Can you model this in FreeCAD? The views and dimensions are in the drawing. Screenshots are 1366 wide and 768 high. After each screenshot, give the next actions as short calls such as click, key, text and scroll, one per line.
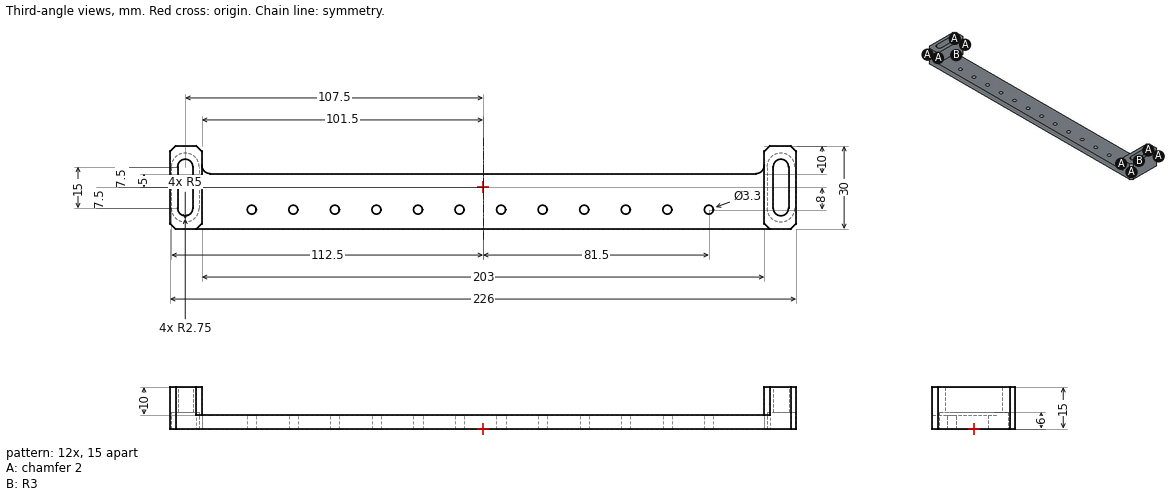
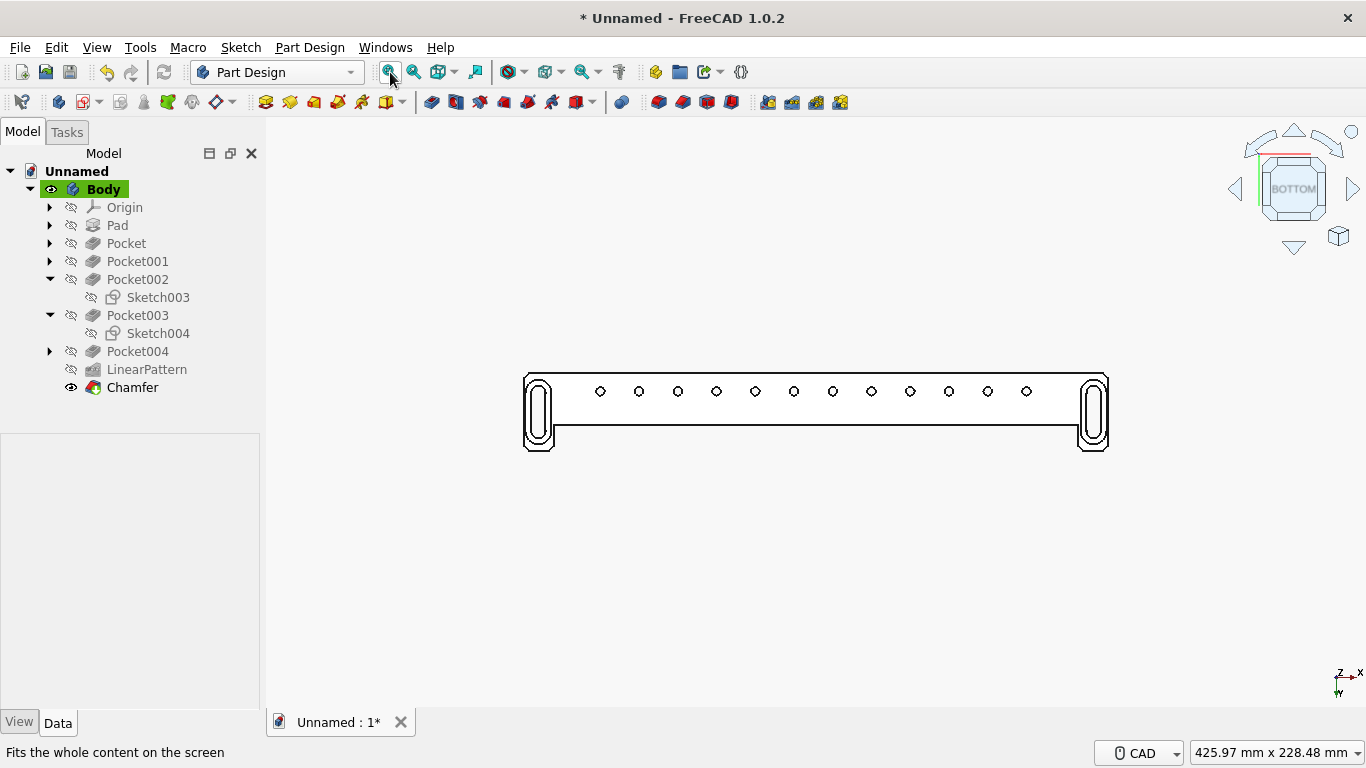
scroll(554, 424, up, 6)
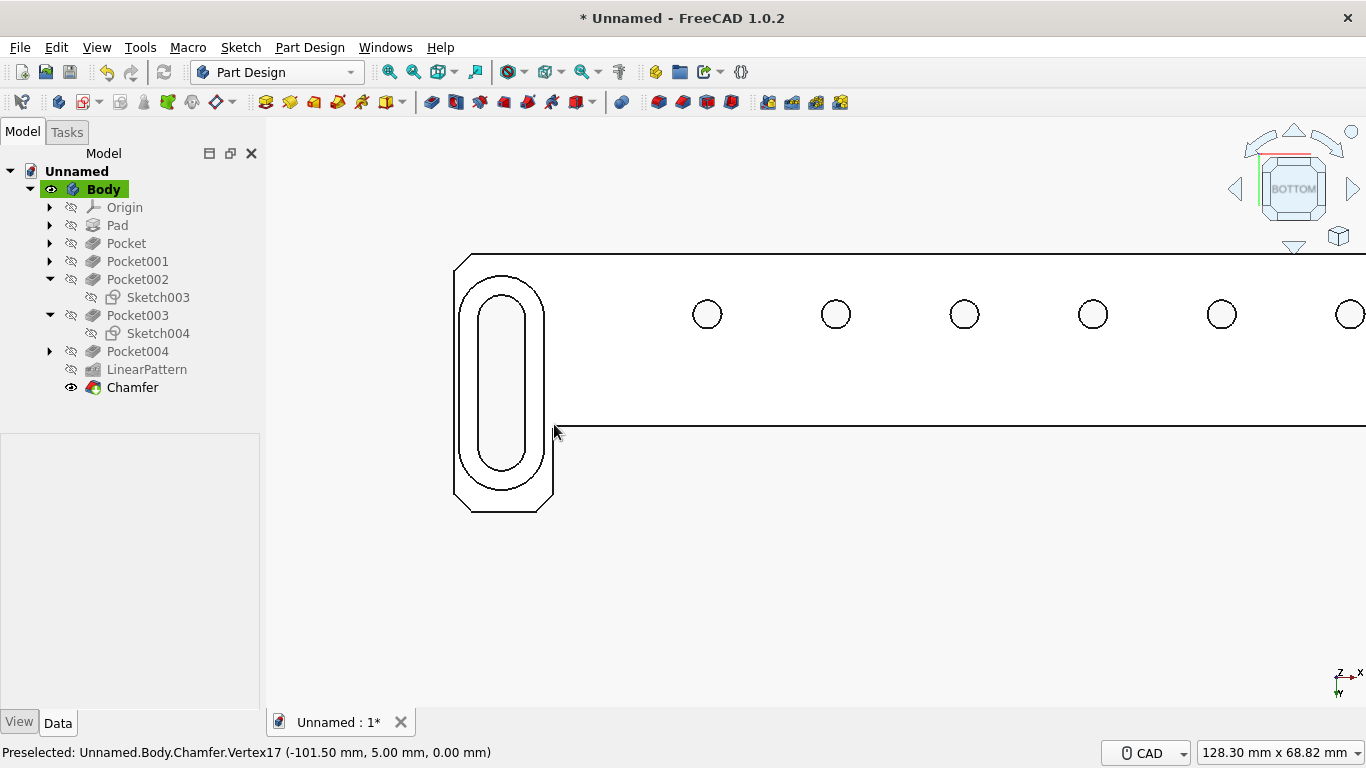
key(v)
key(f)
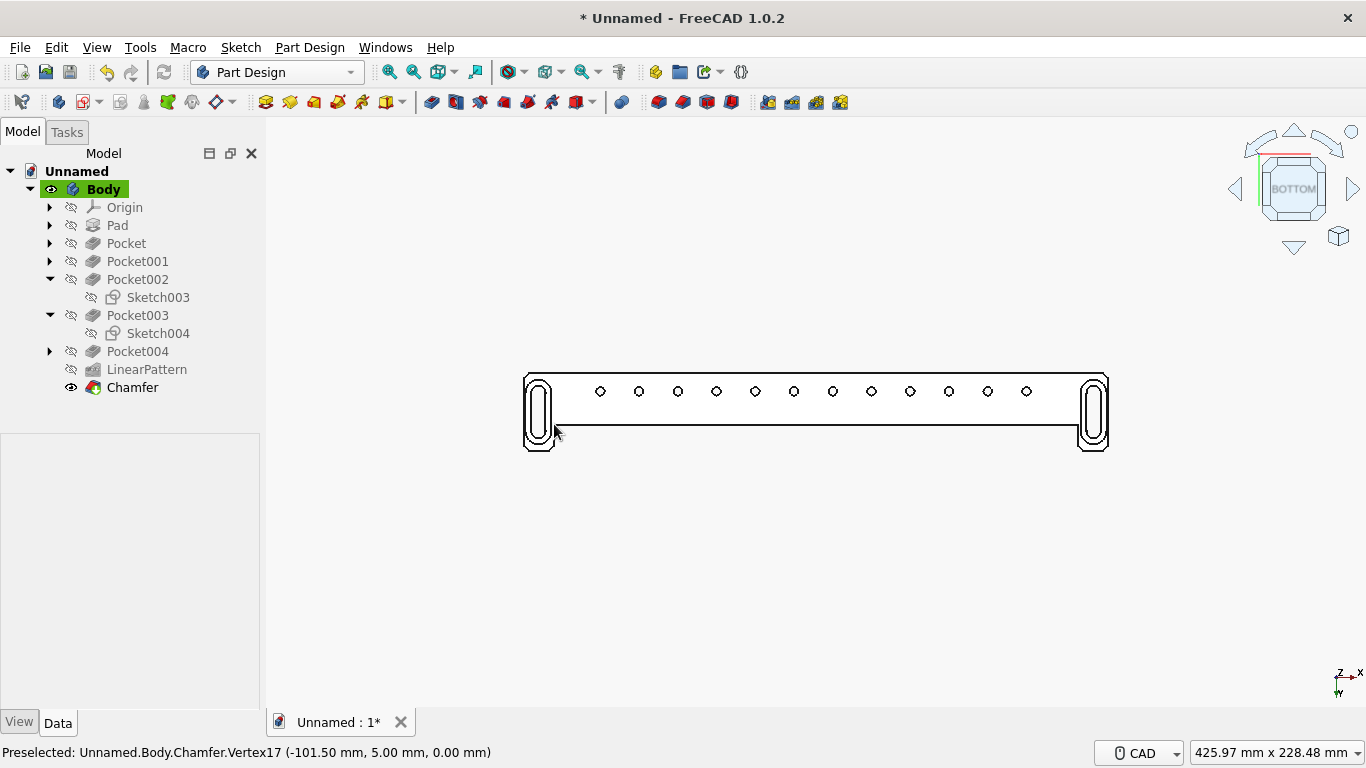
key(4)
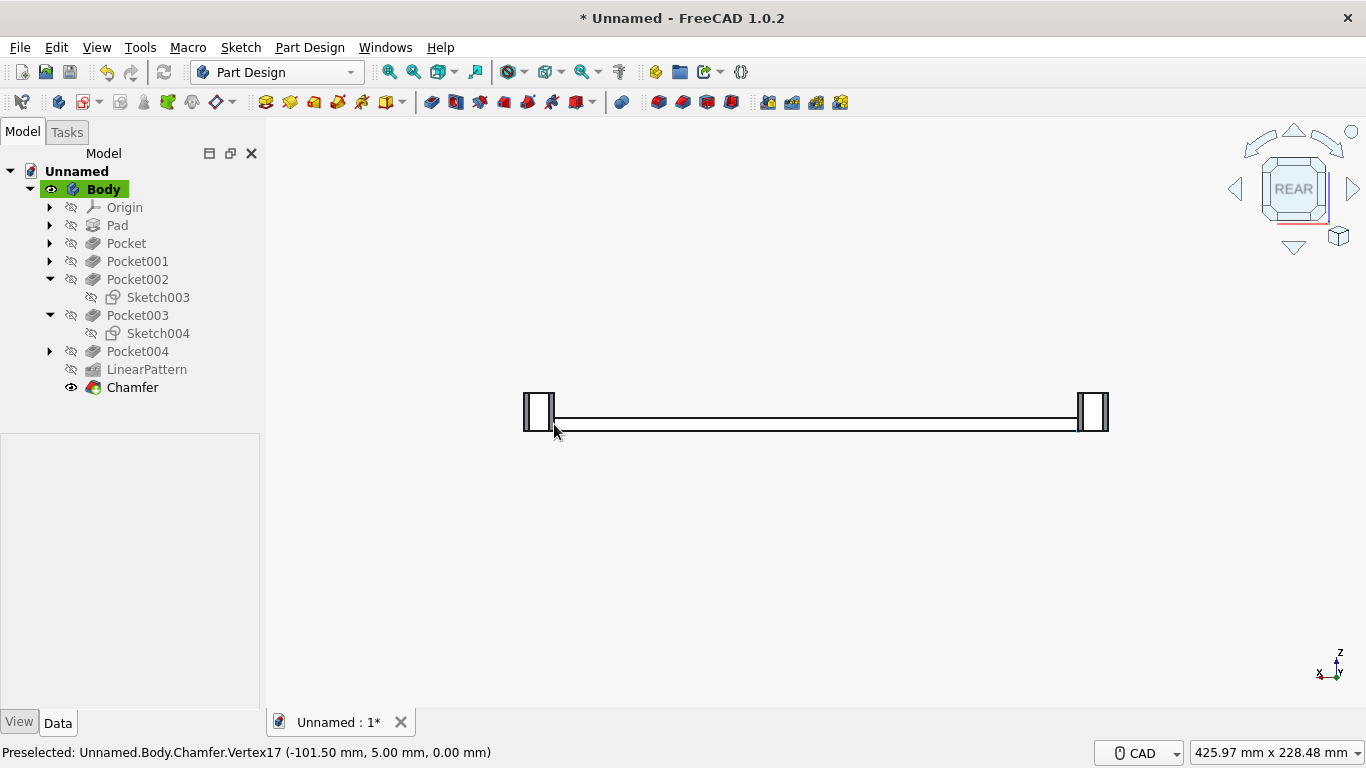
scroll(1078, 424, up, 6)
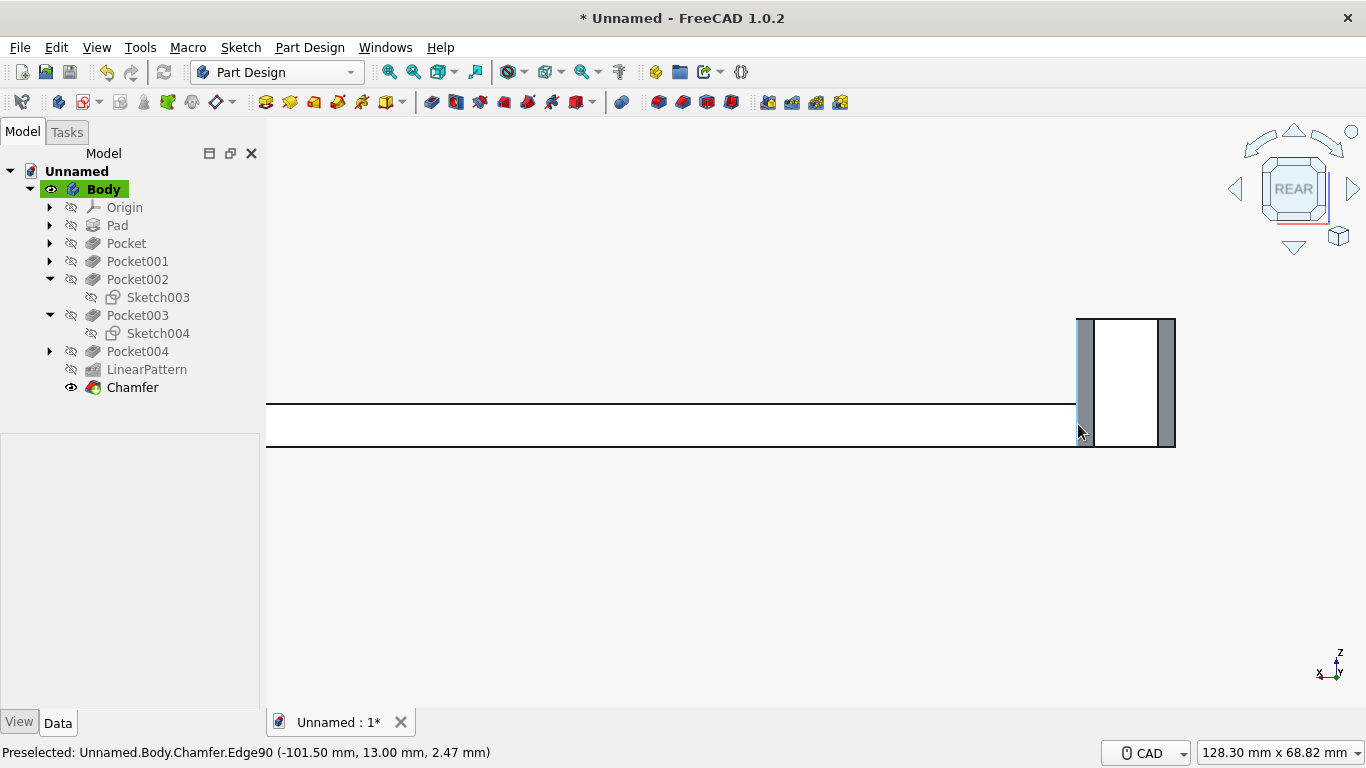
key(v)
key(f)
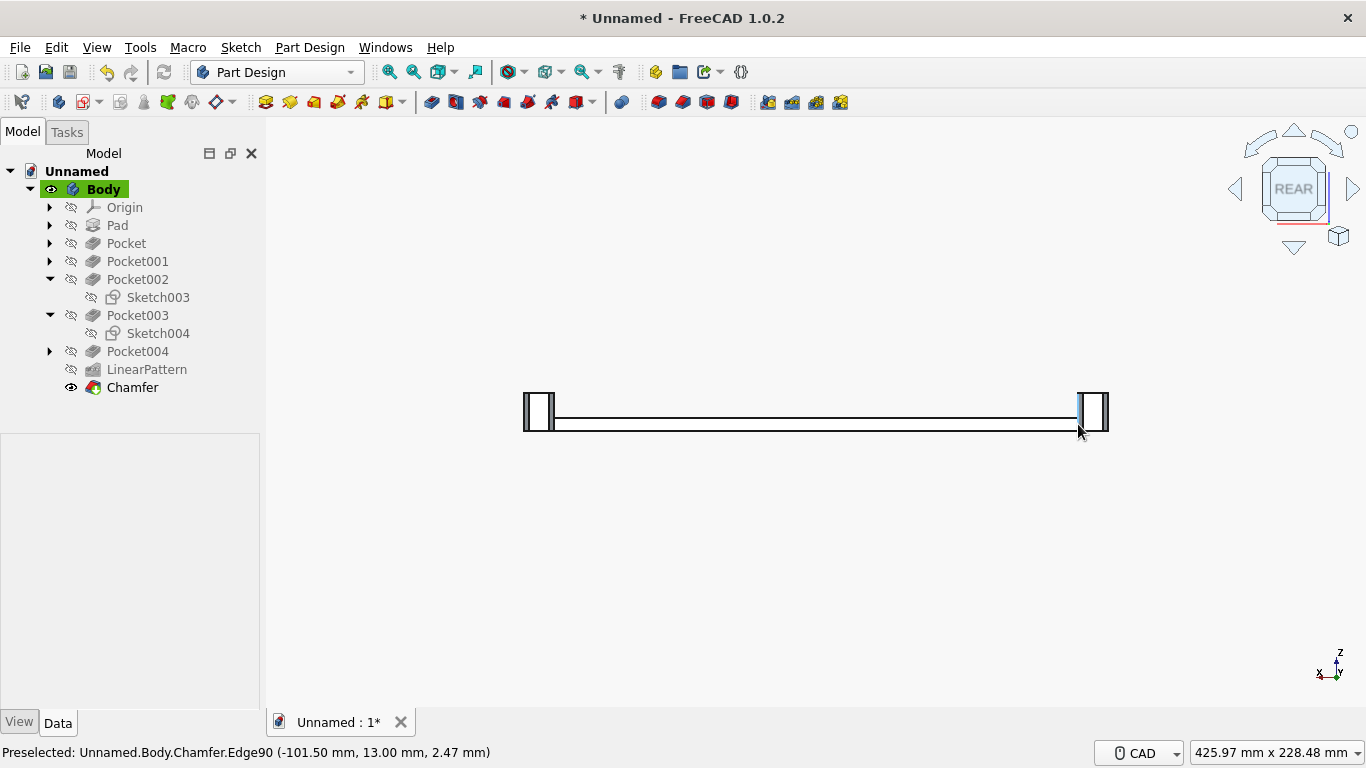
key(6)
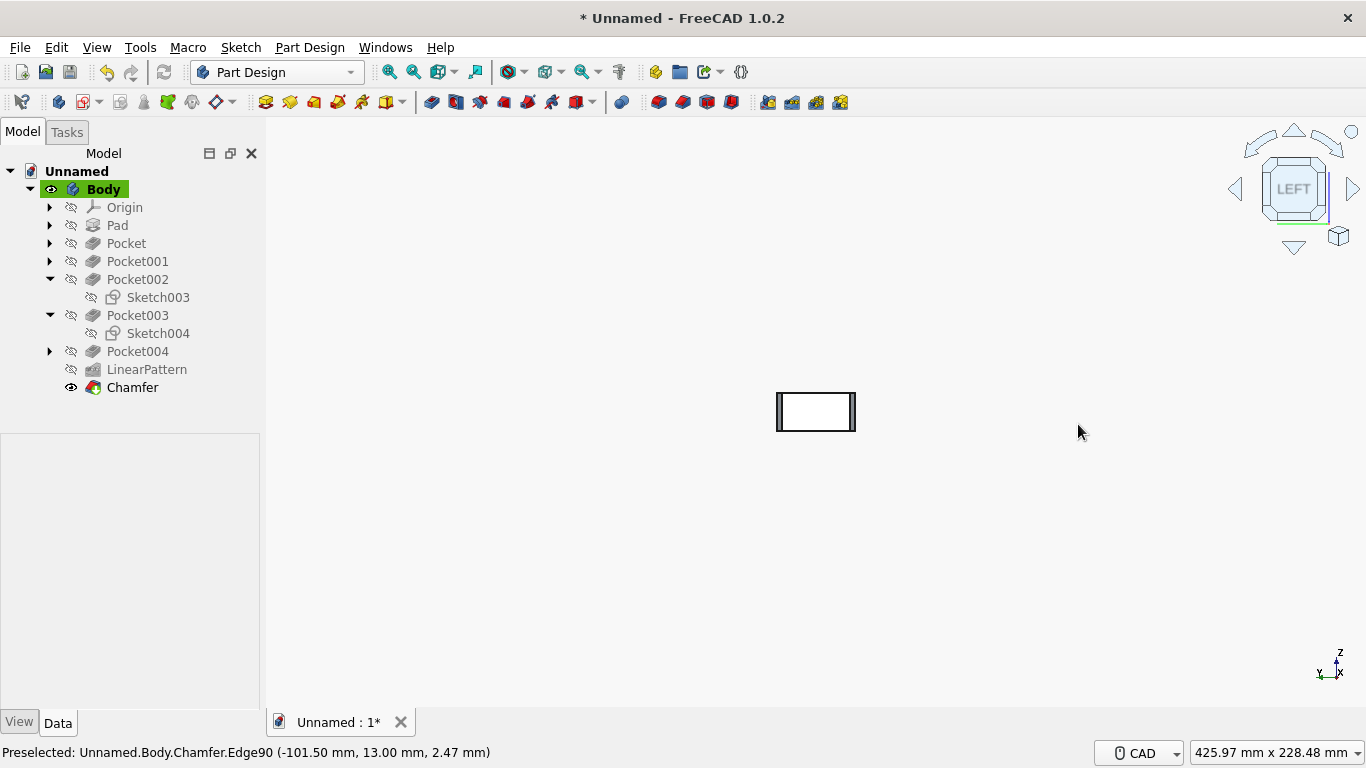
key(v)
key(f)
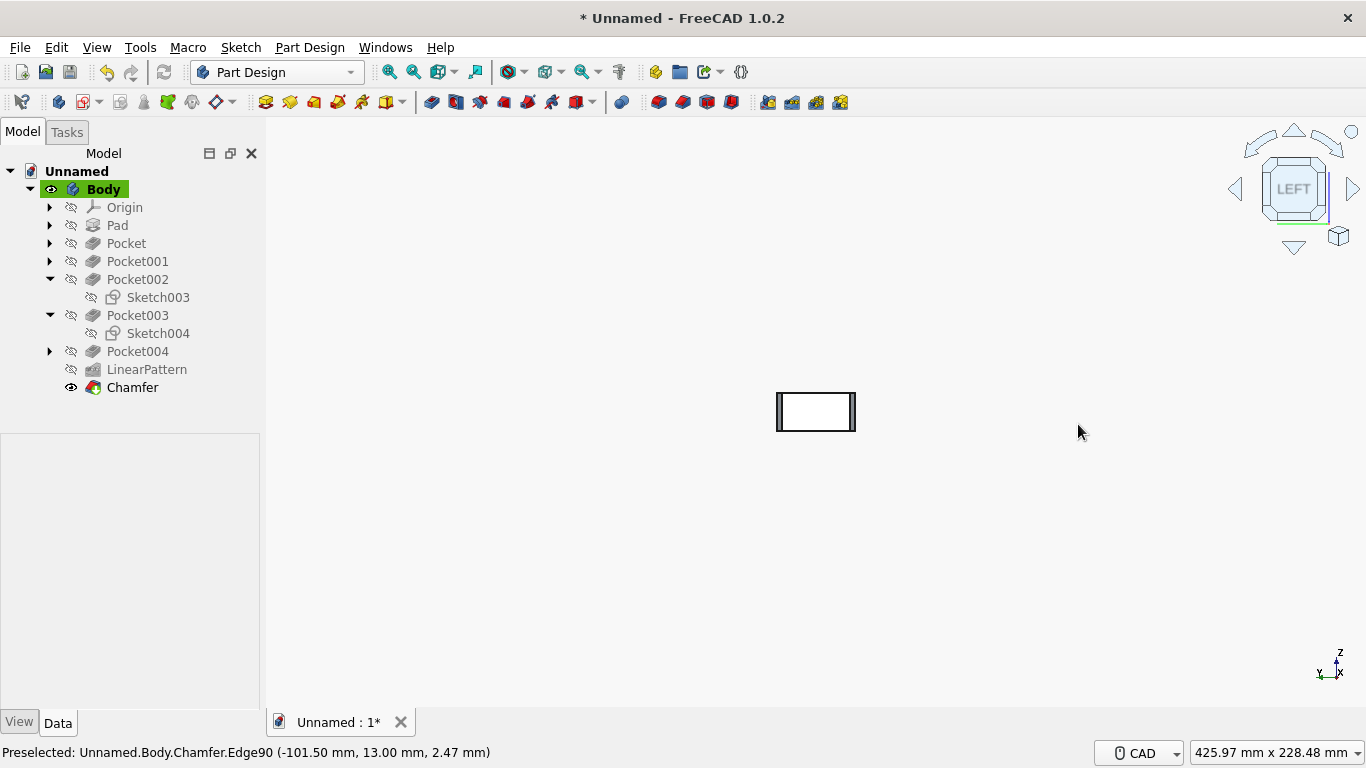
scroll(803, 424, up, 6)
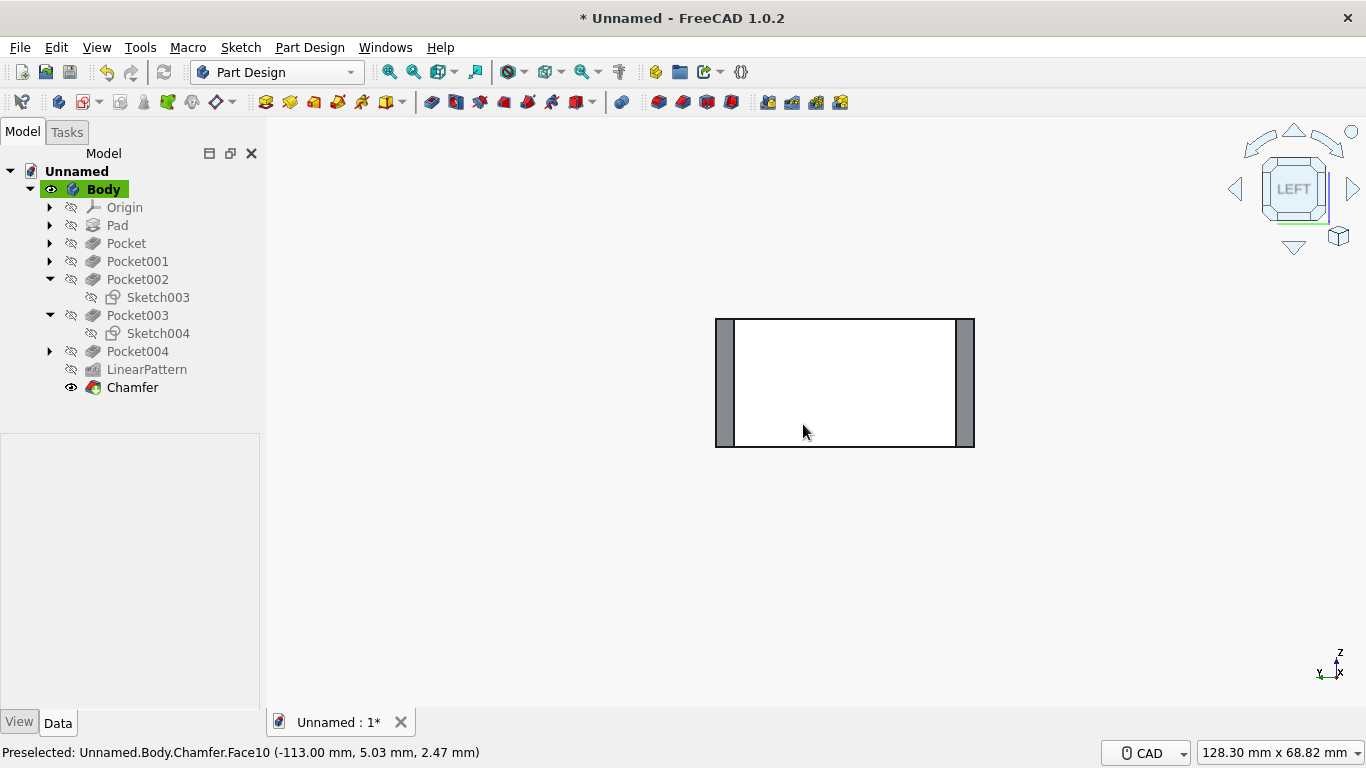
key(v)
key(f)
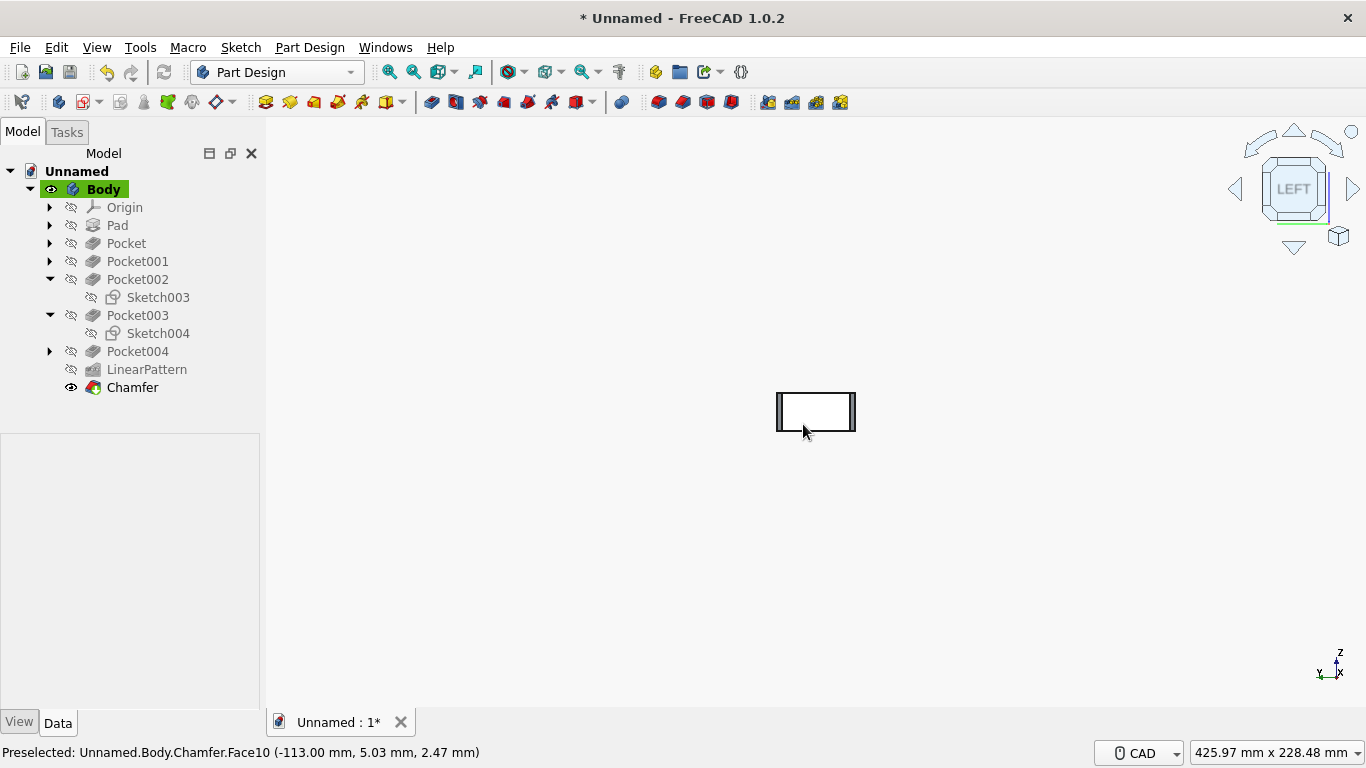
key(v)
key(3)